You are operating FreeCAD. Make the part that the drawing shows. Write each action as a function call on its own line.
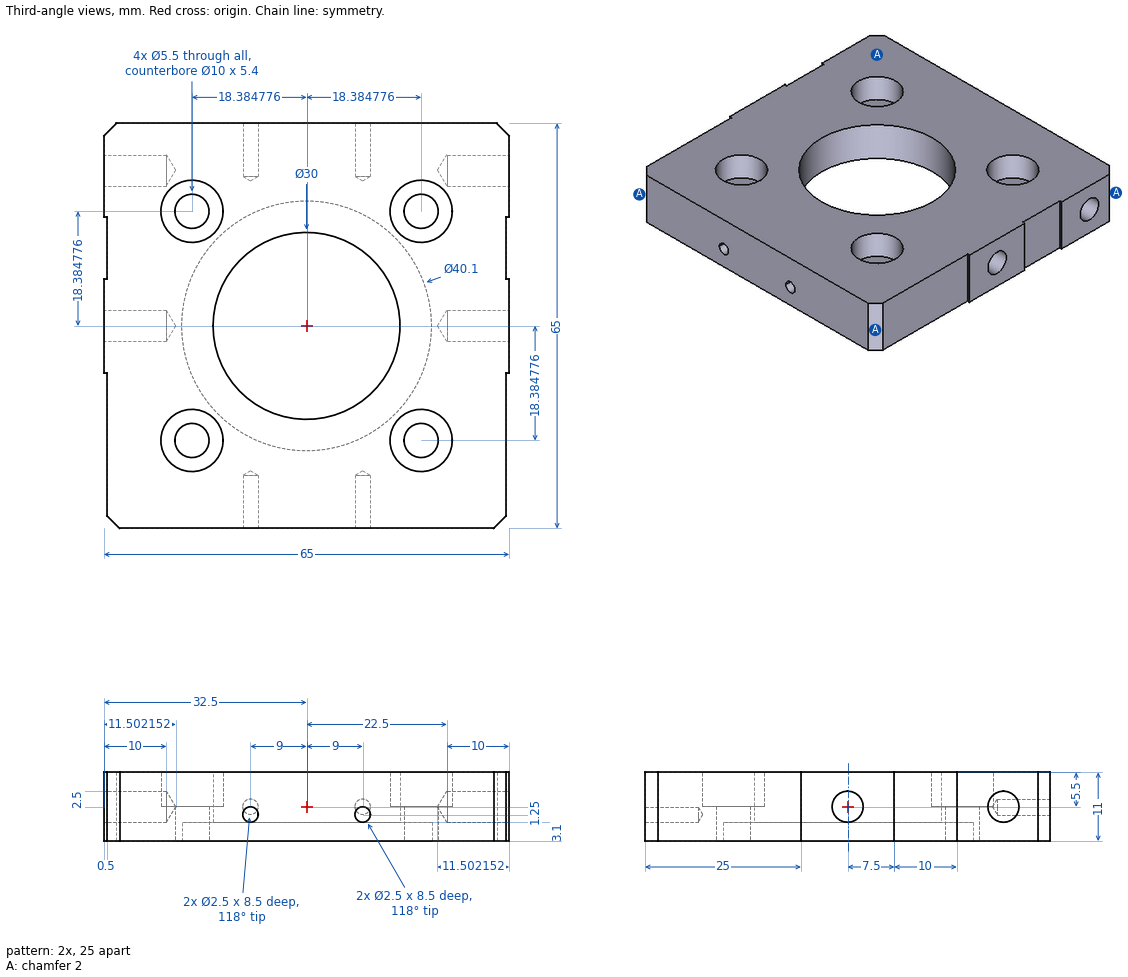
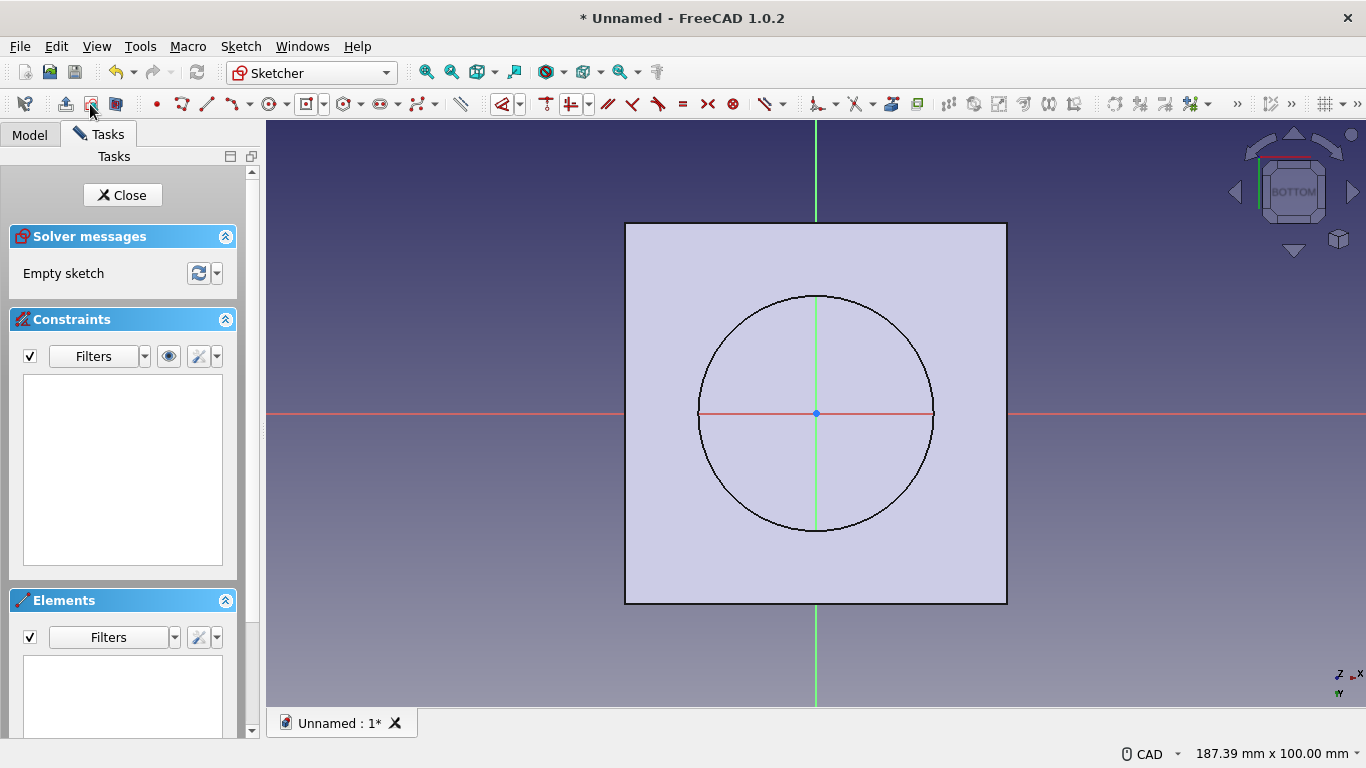
click(116, 104)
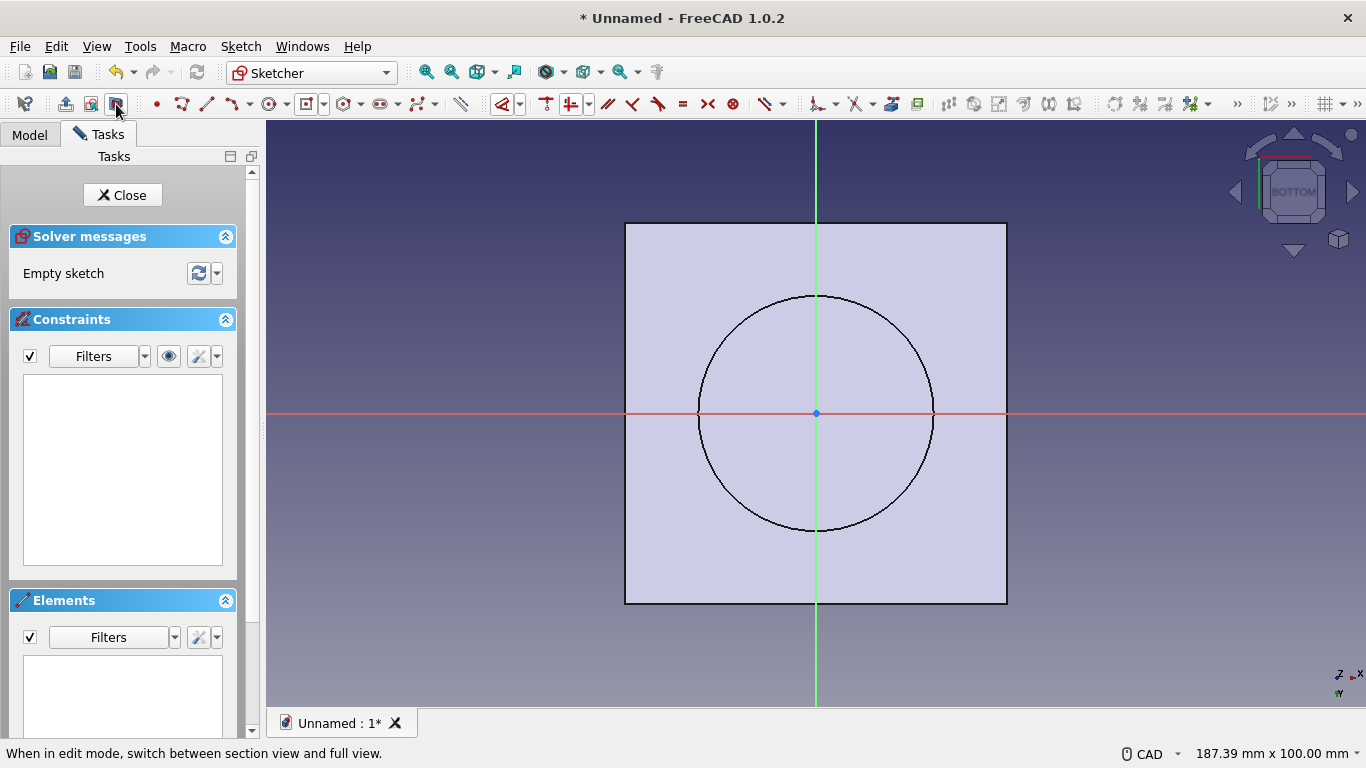
scroll(872, 414, up, 4)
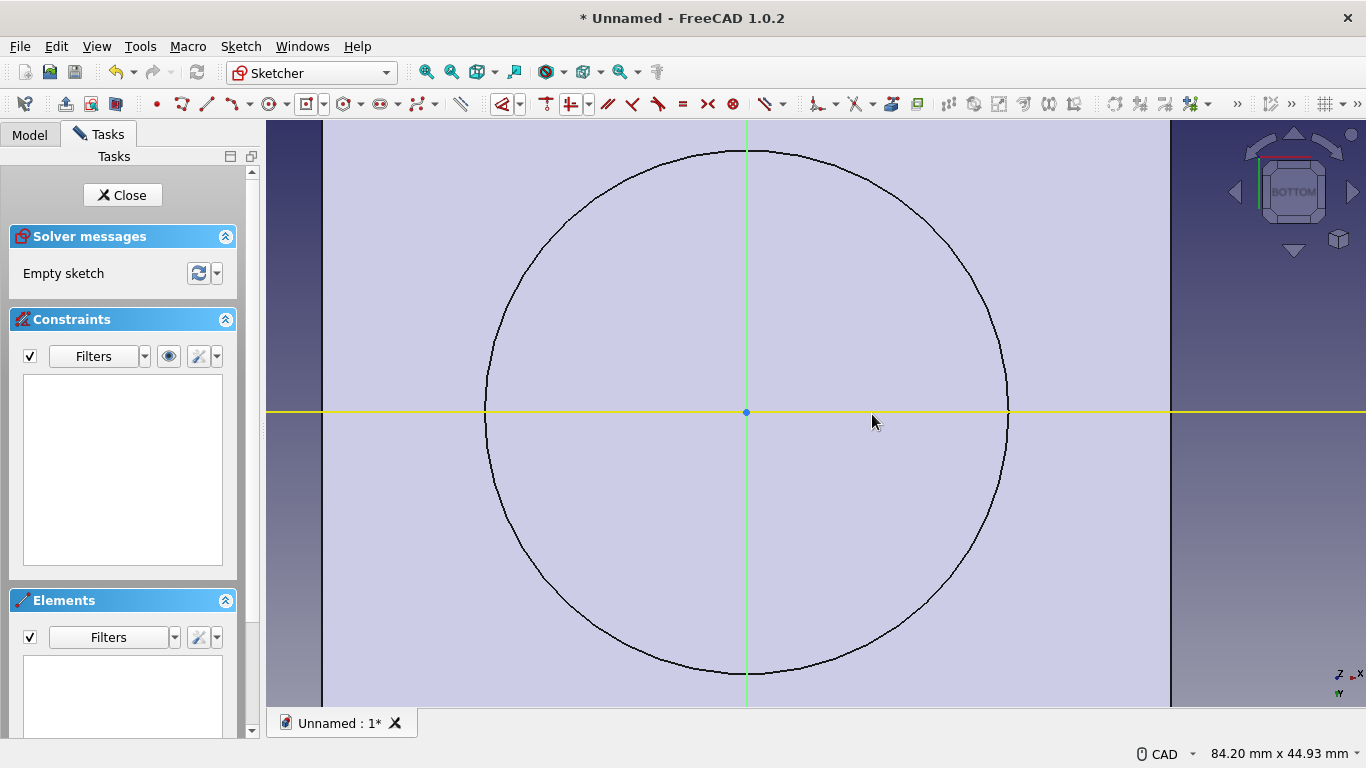
click(268, 104)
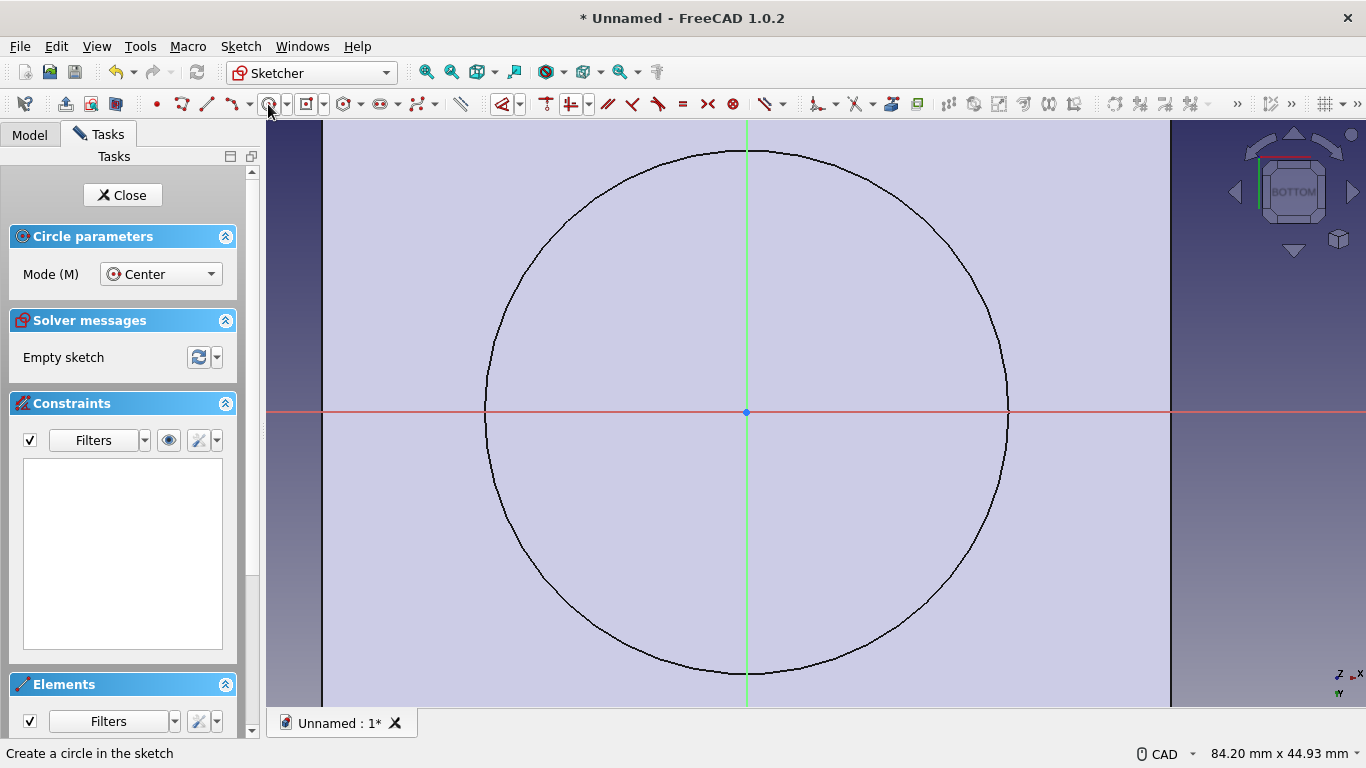
click(747, 412)
click(885, 274)
key(Escape)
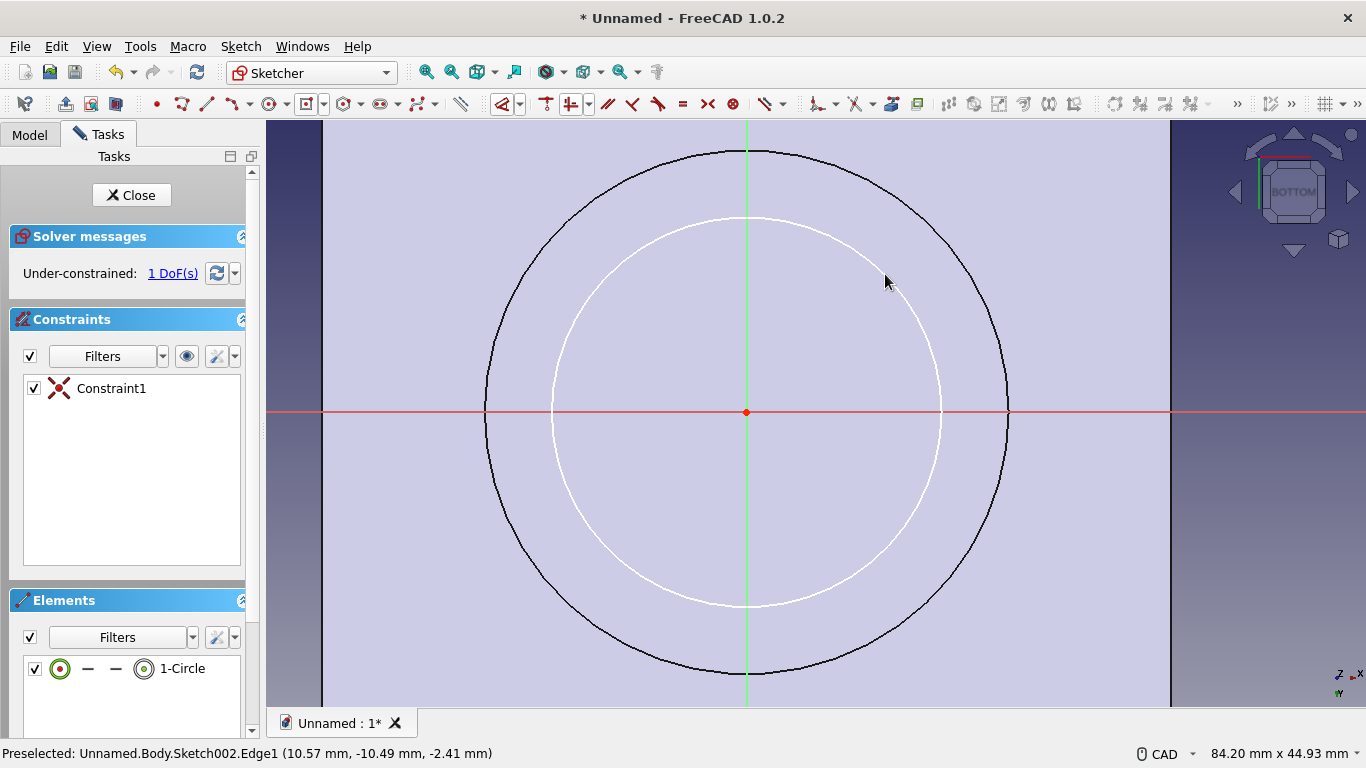
click(884, 274)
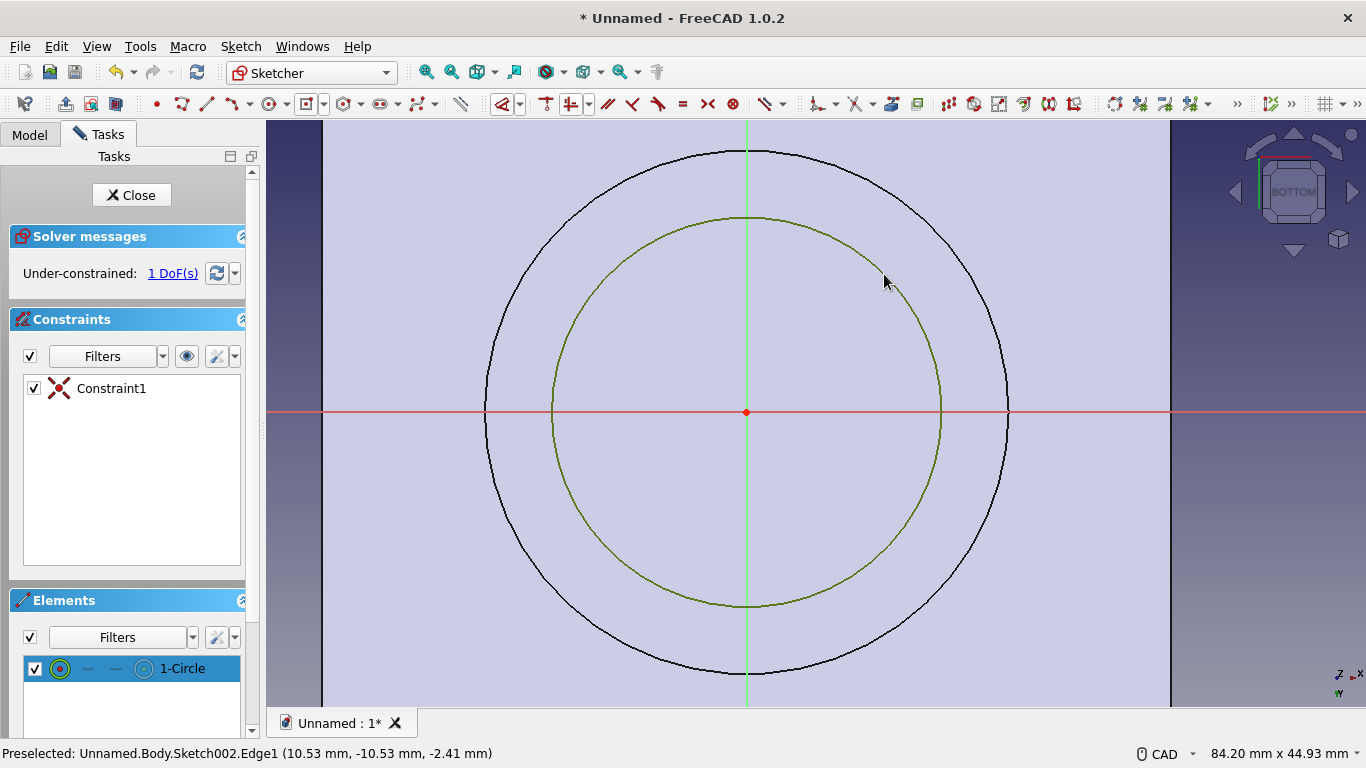
click(520, 104)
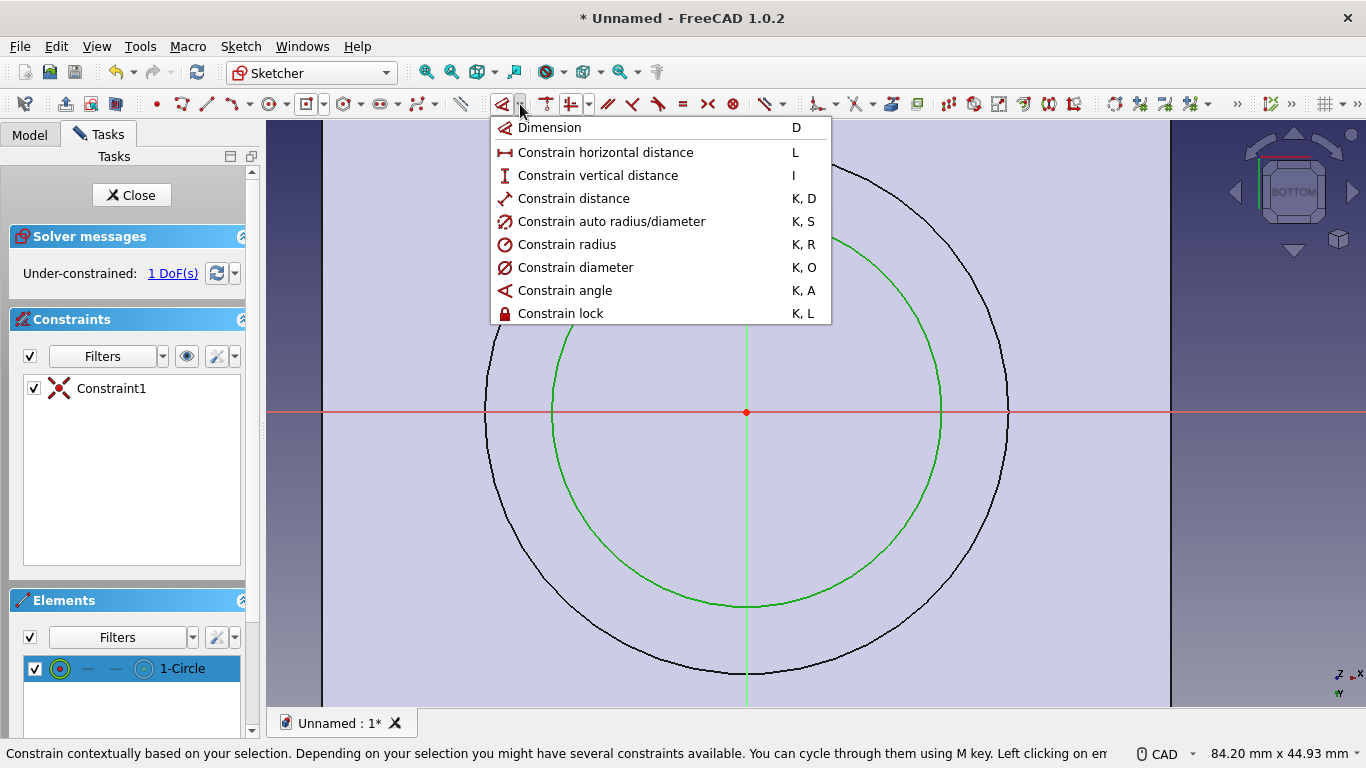
click(661, 268)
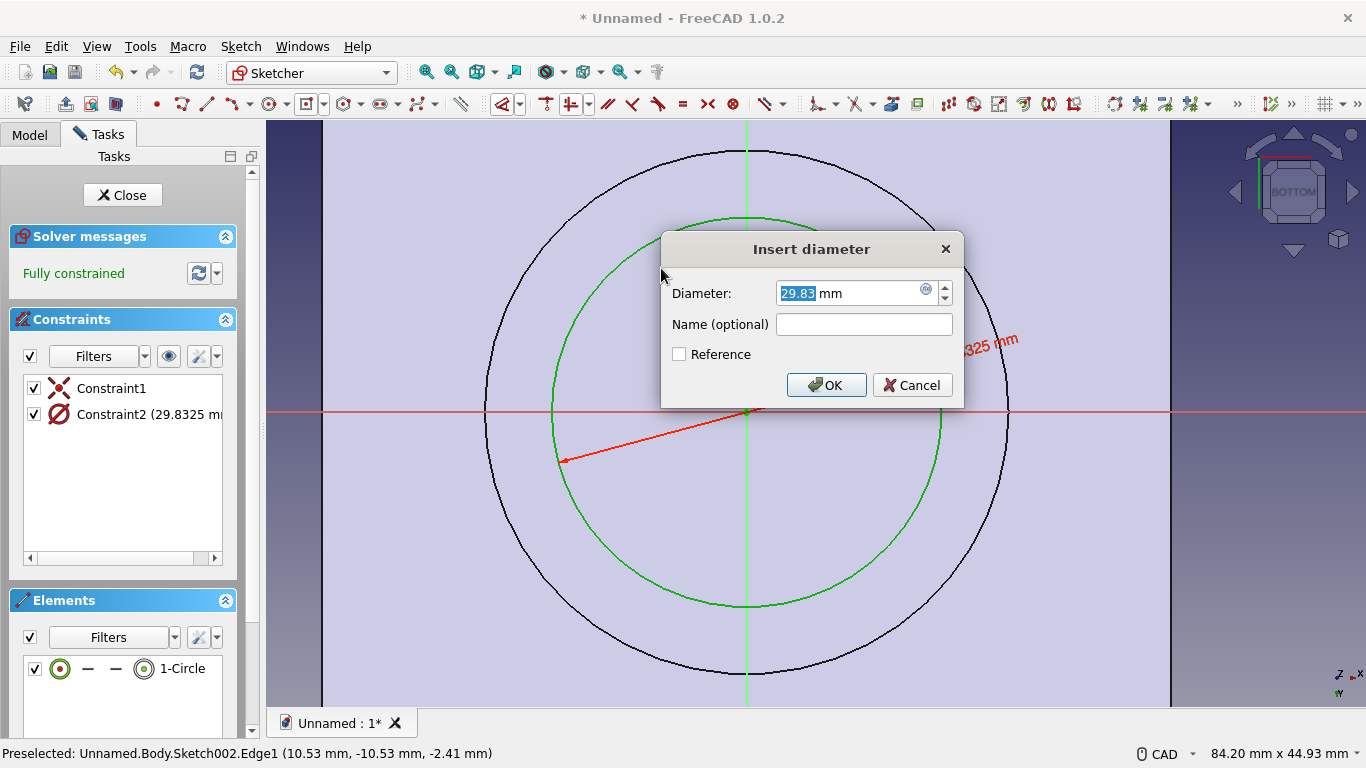
text(30)
key(Return)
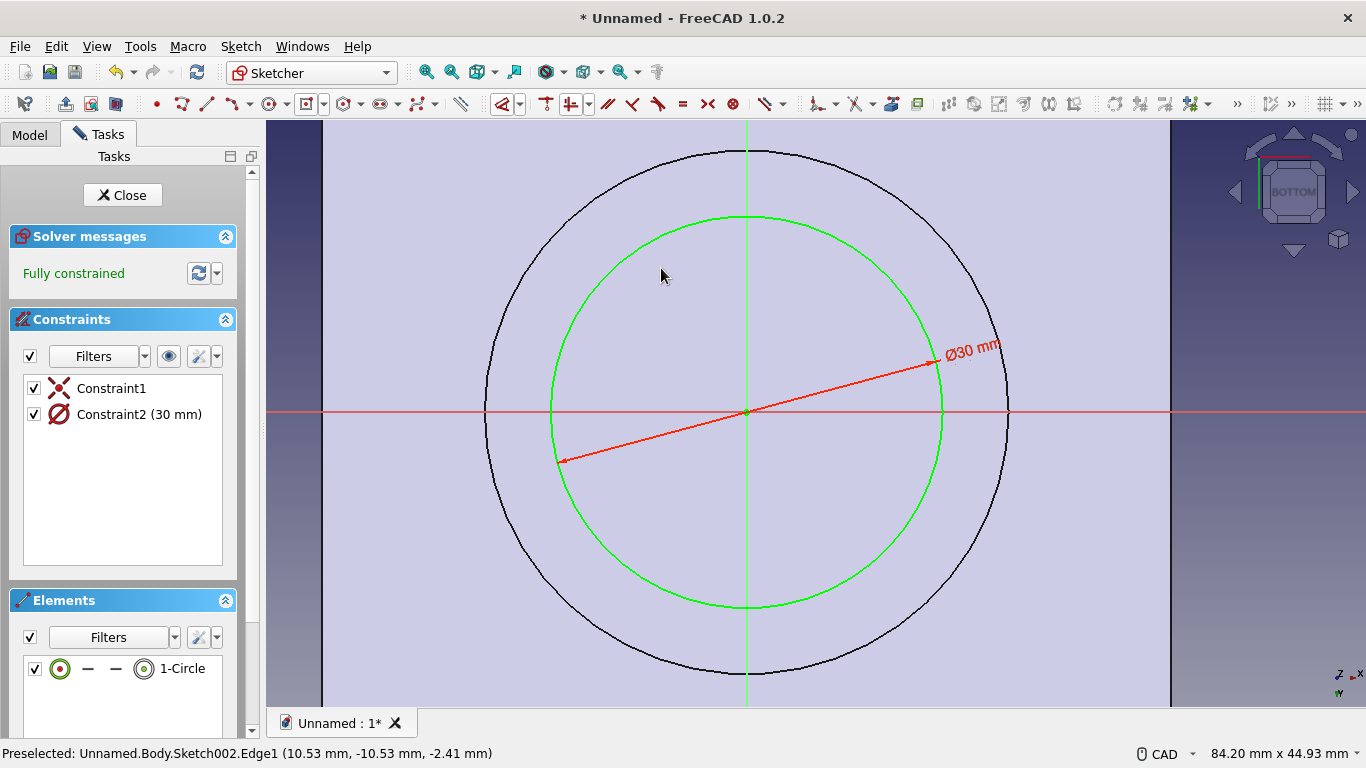
click(123, 195)